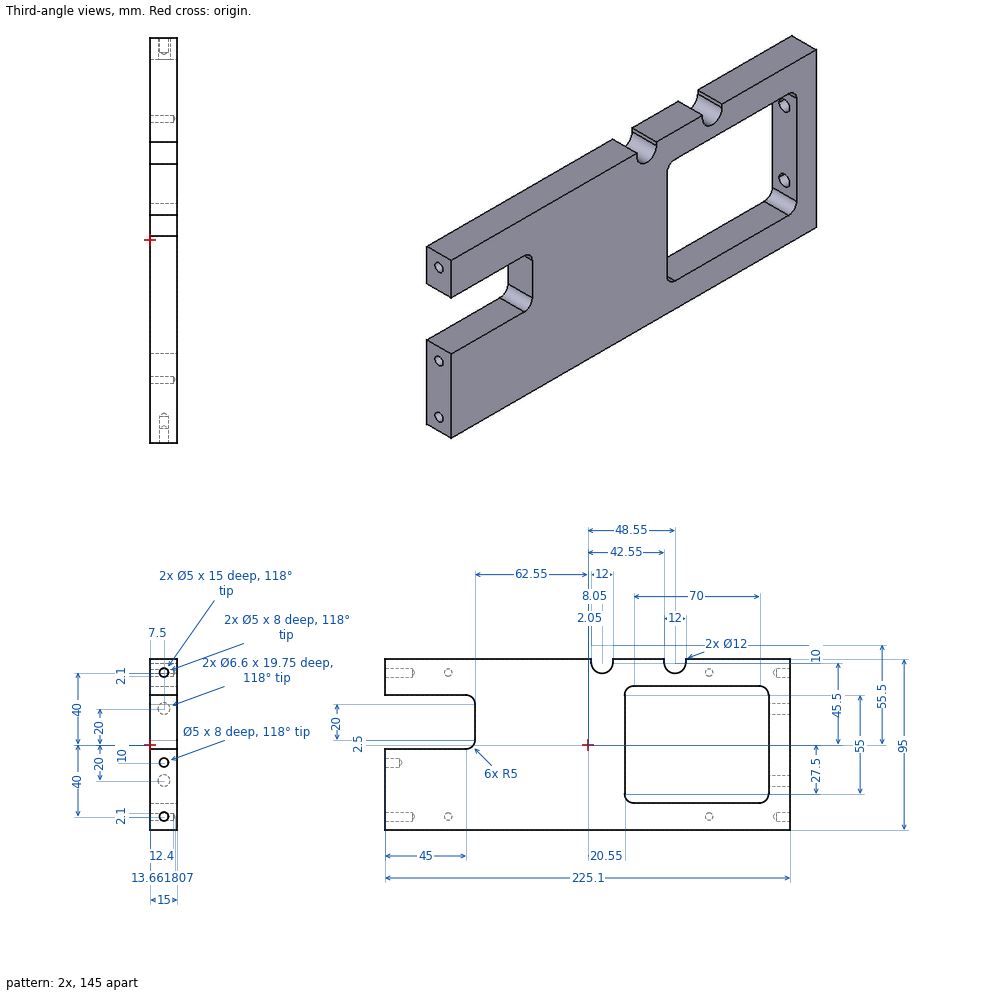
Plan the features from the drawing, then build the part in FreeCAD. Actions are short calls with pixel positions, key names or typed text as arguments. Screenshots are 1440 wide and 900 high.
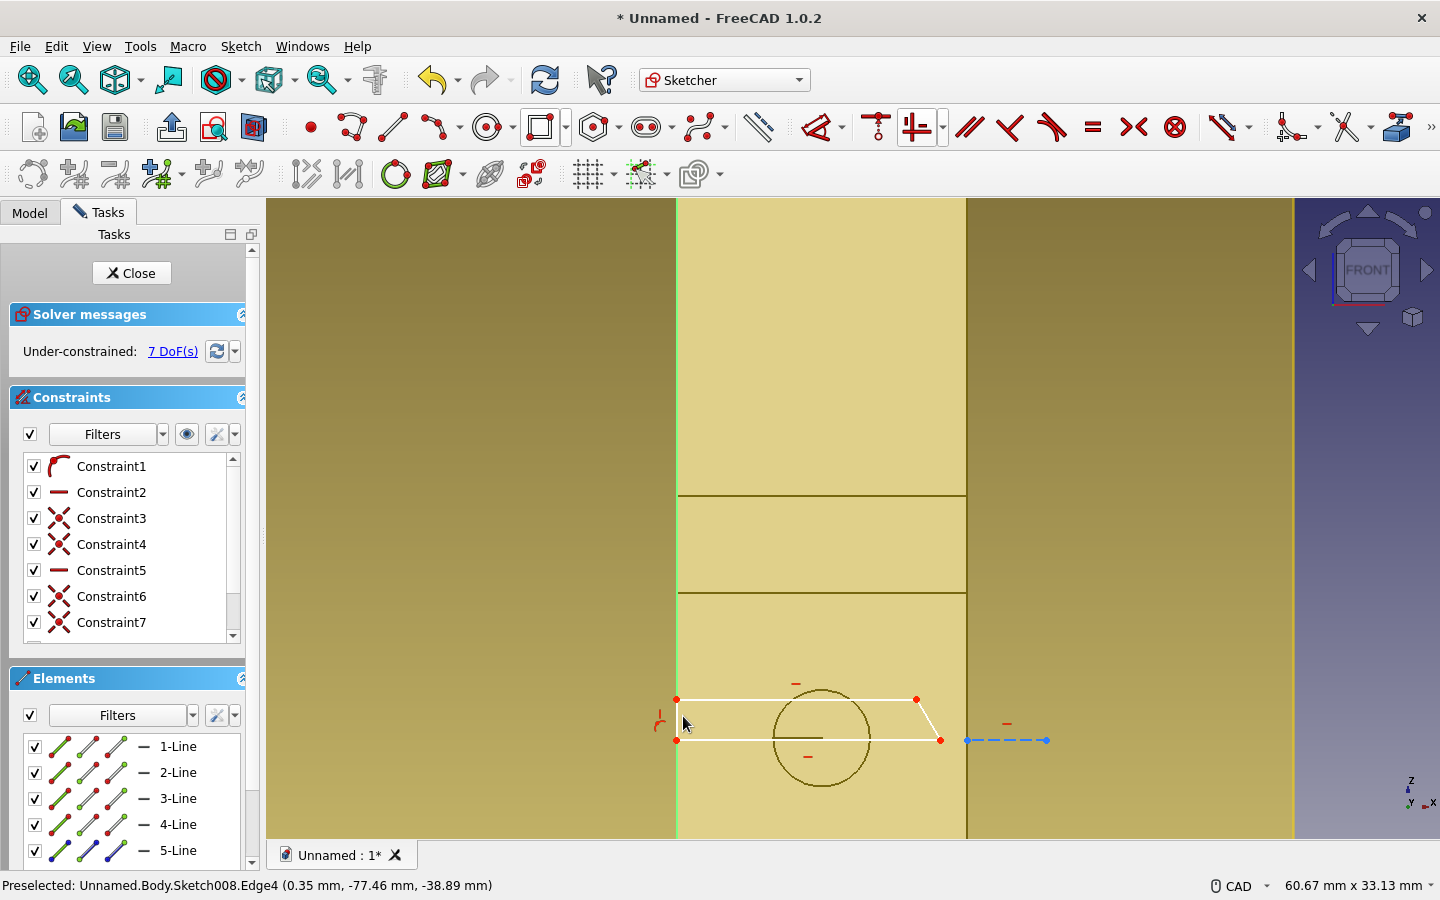
click(816, 128)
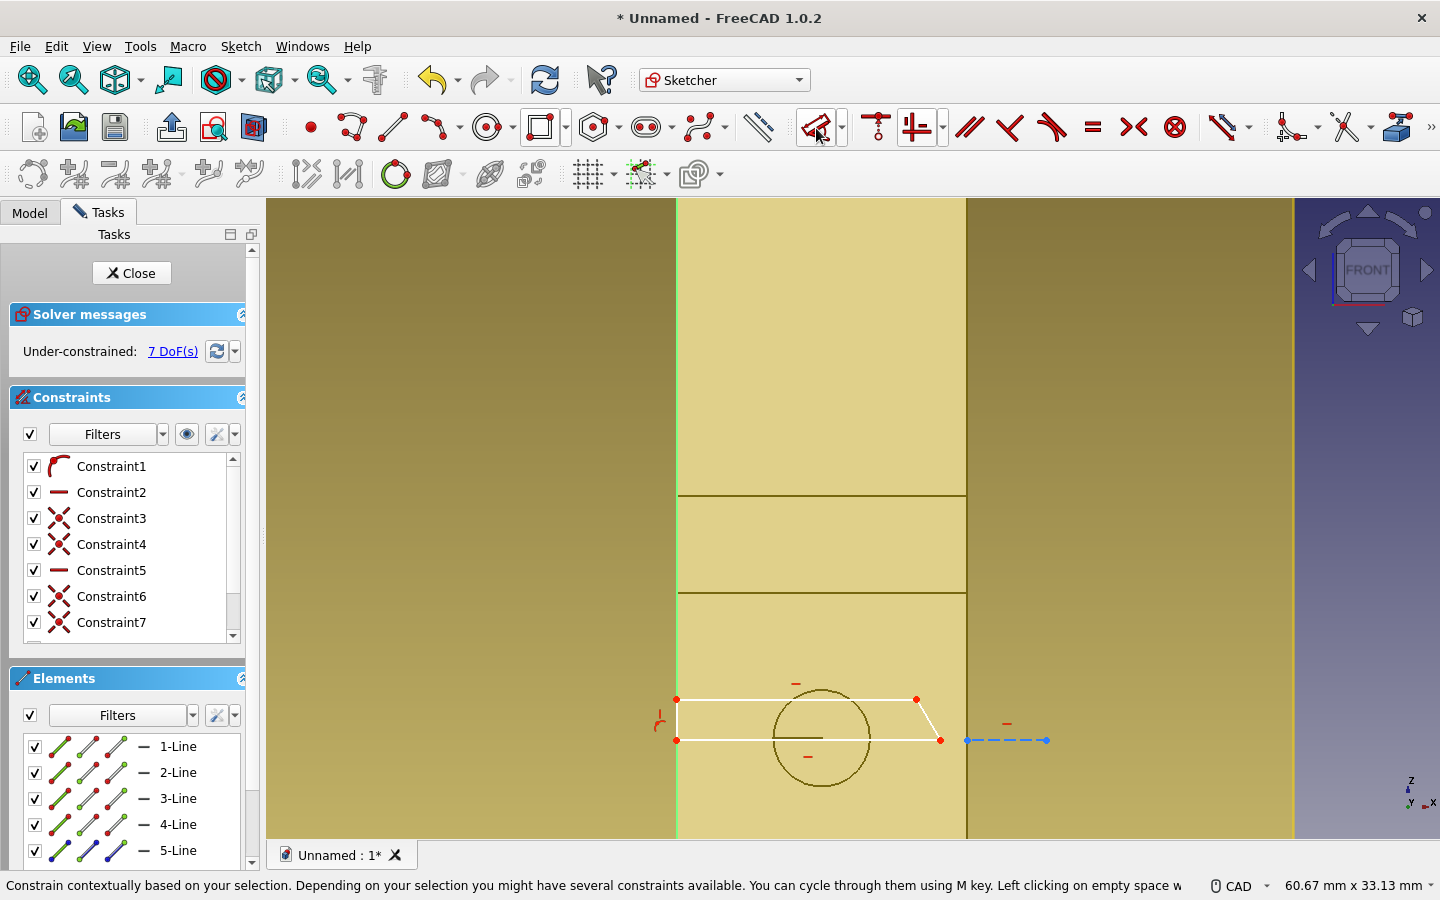
click(677, 728)
click(643, 720)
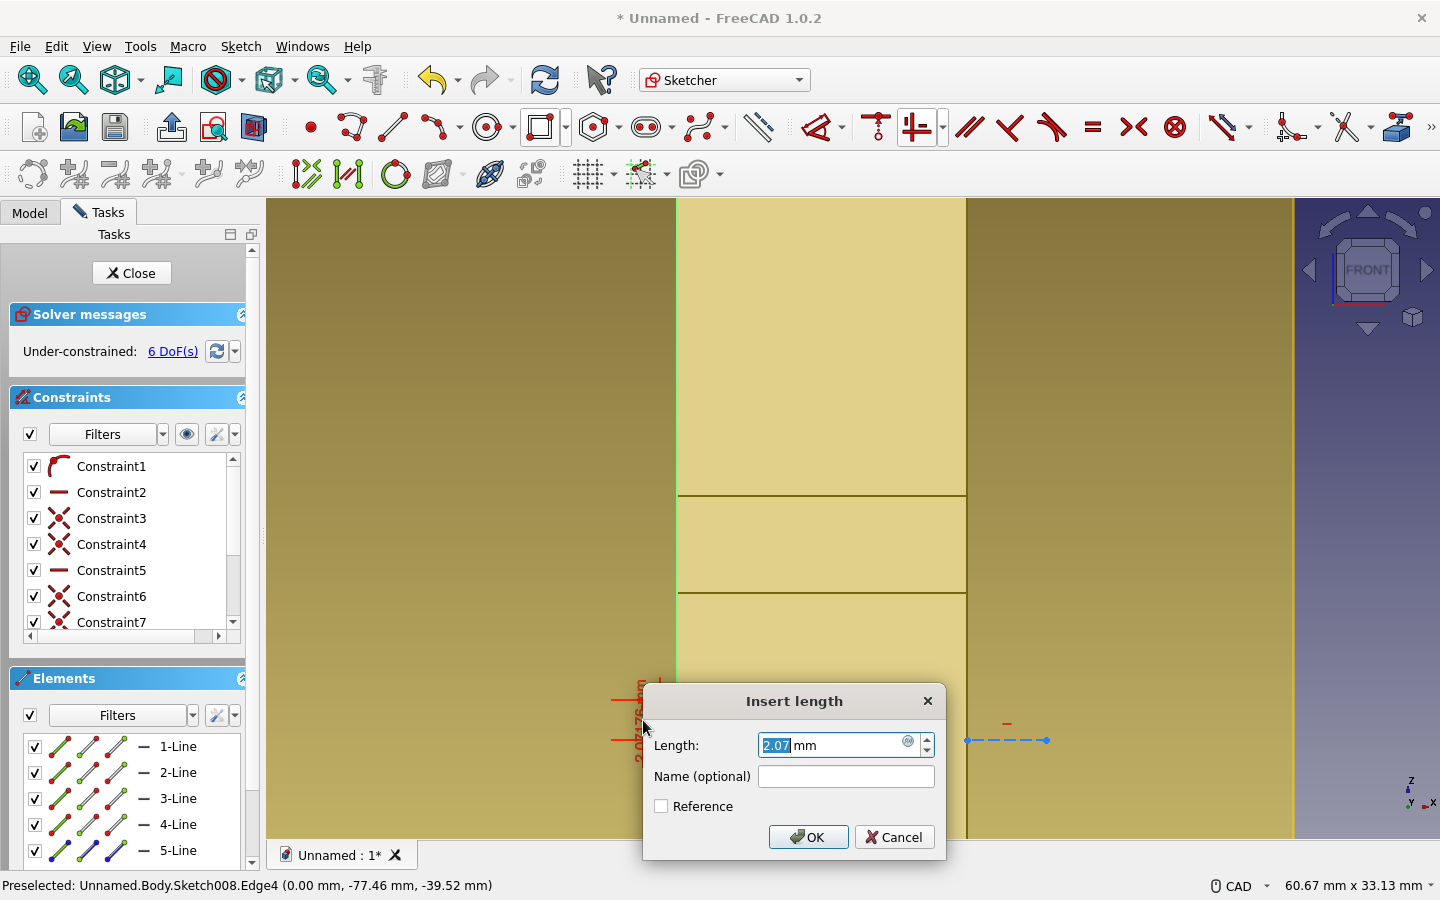
text(2.1)
key(Return)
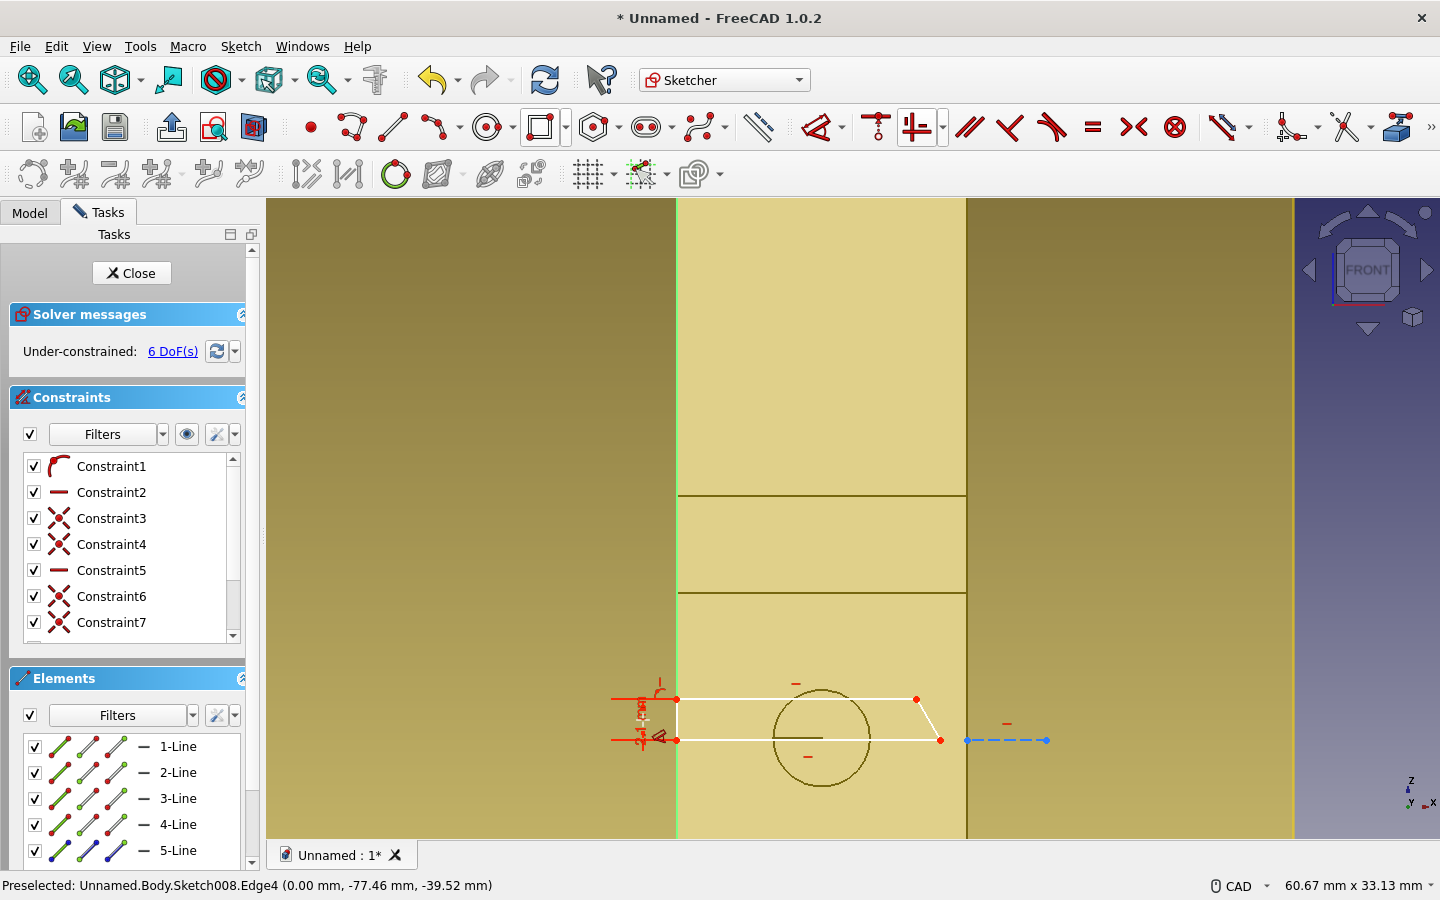
click(941, 740)
click(643, 483)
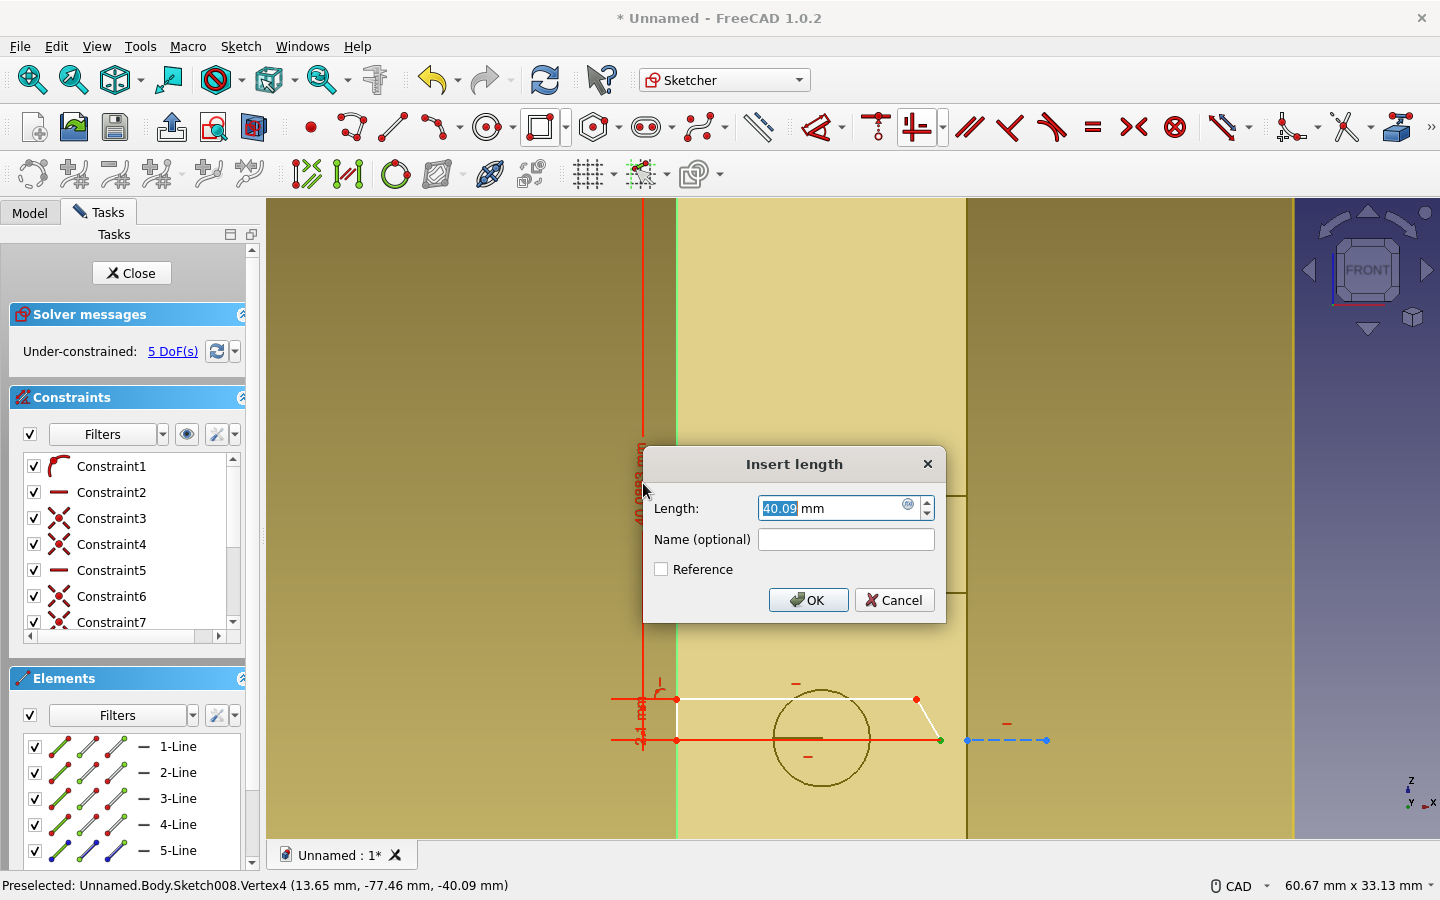
text(40)
key(Return)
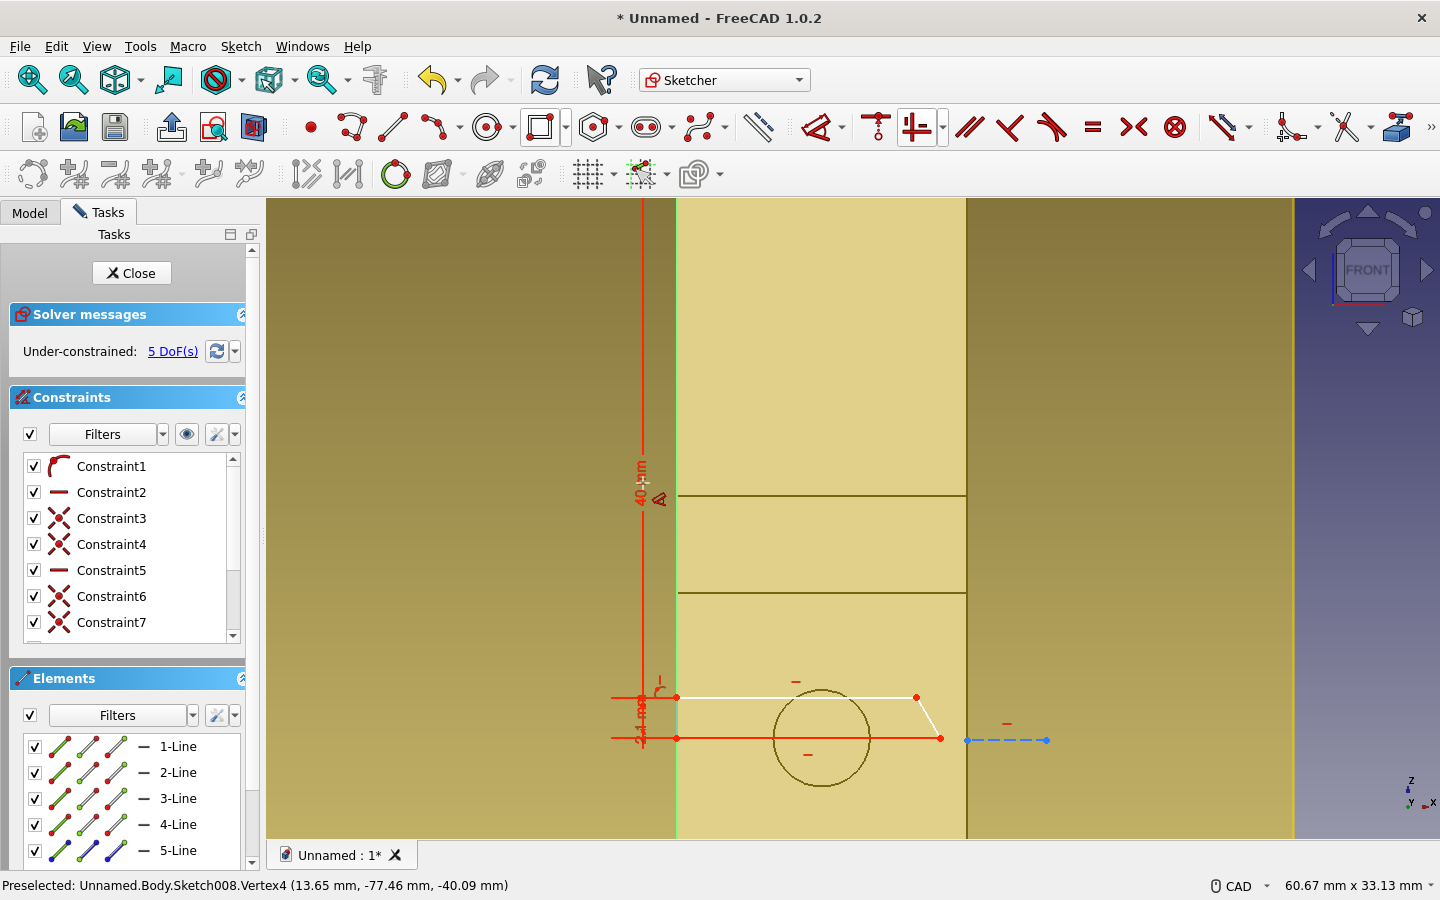
click(968, 740)
click(643, 365)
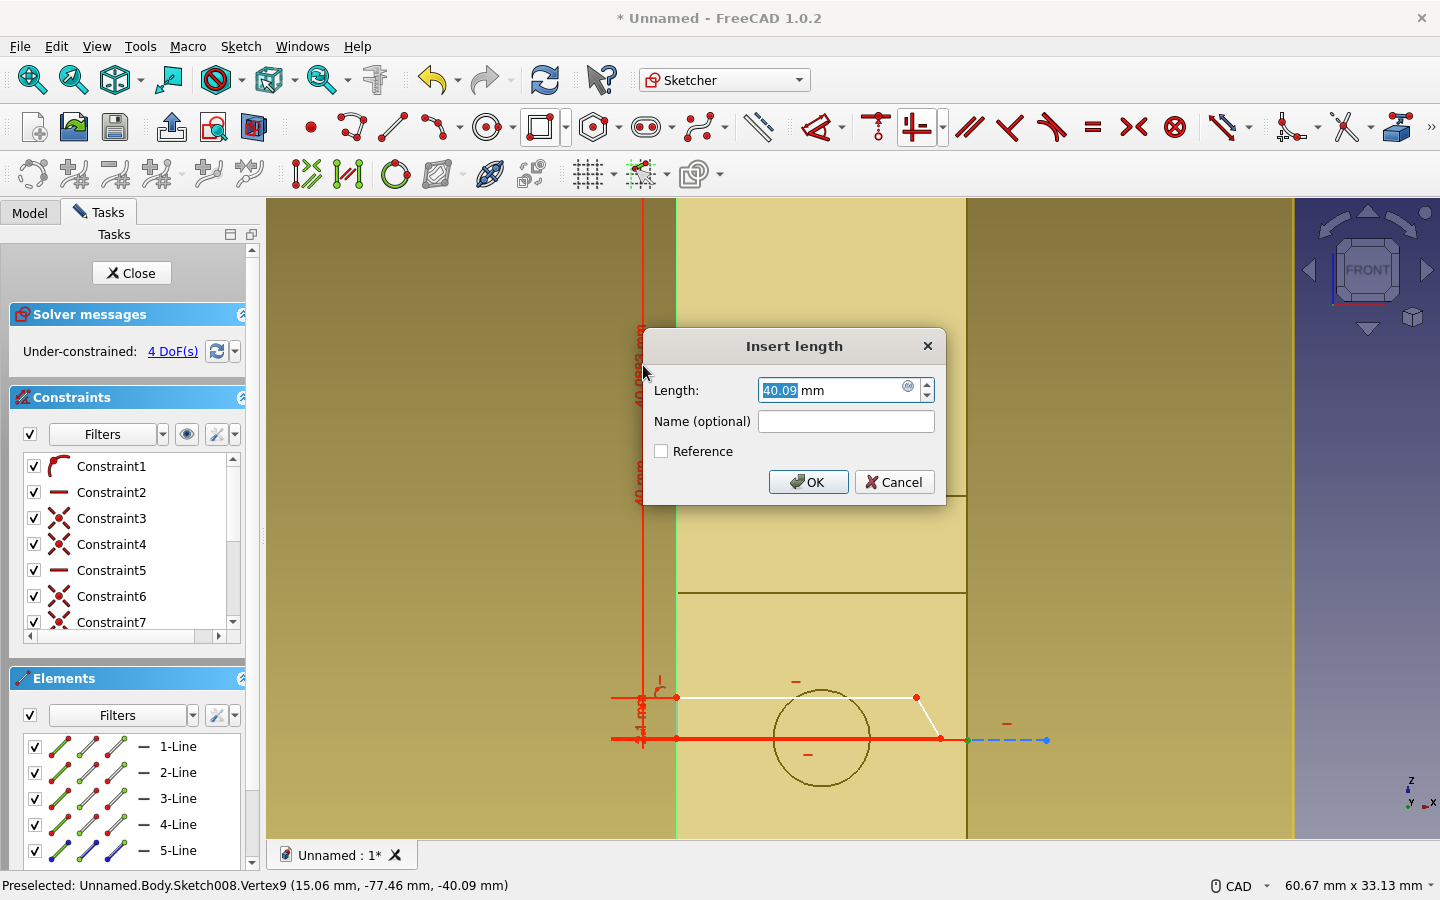
text(40)
key(Return)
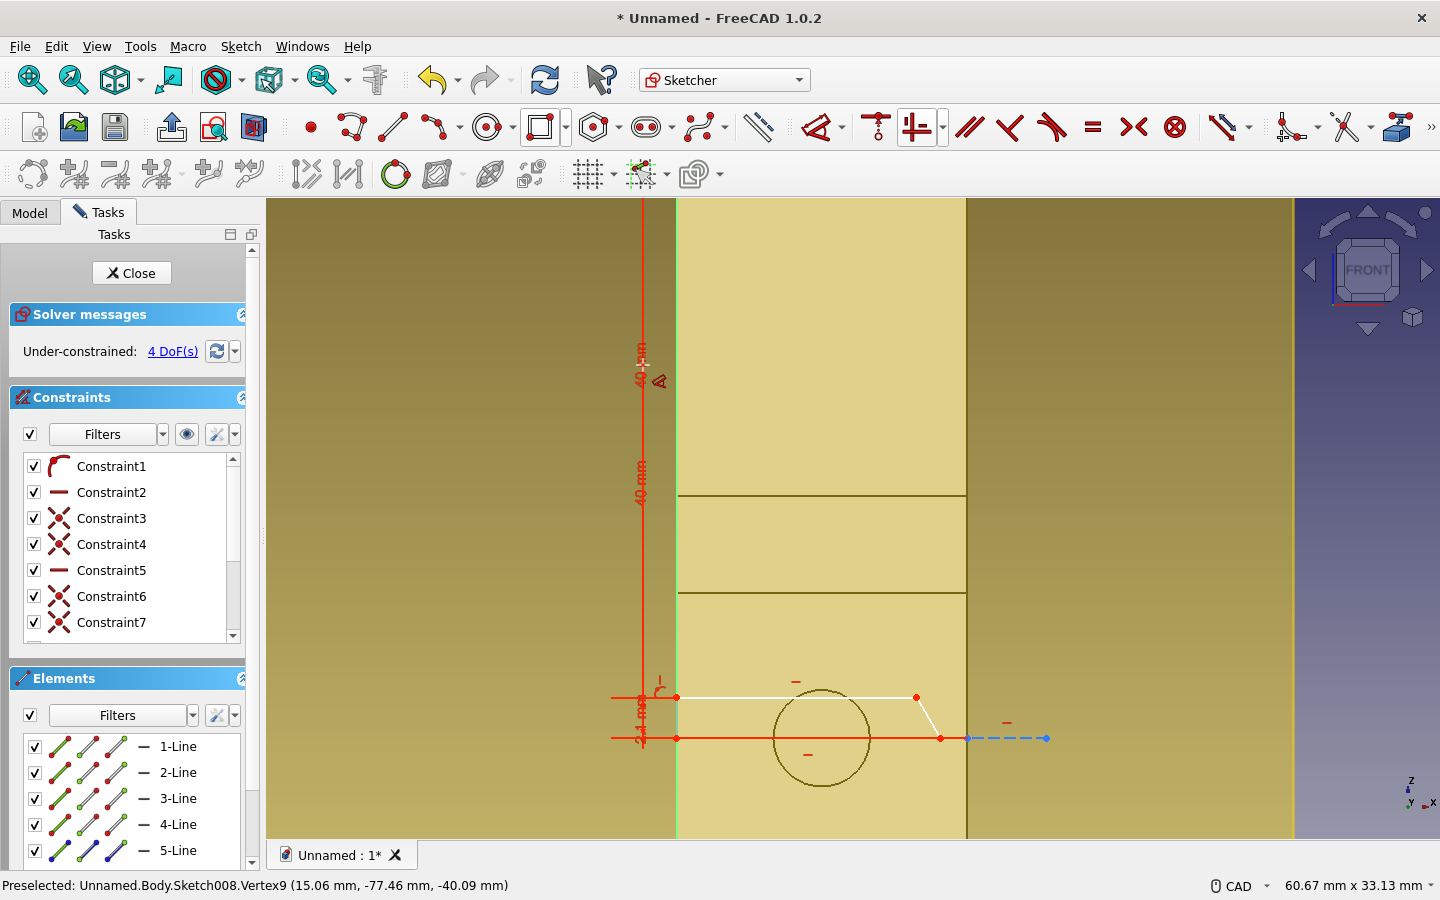
click(749, 698)
click(797, 664)